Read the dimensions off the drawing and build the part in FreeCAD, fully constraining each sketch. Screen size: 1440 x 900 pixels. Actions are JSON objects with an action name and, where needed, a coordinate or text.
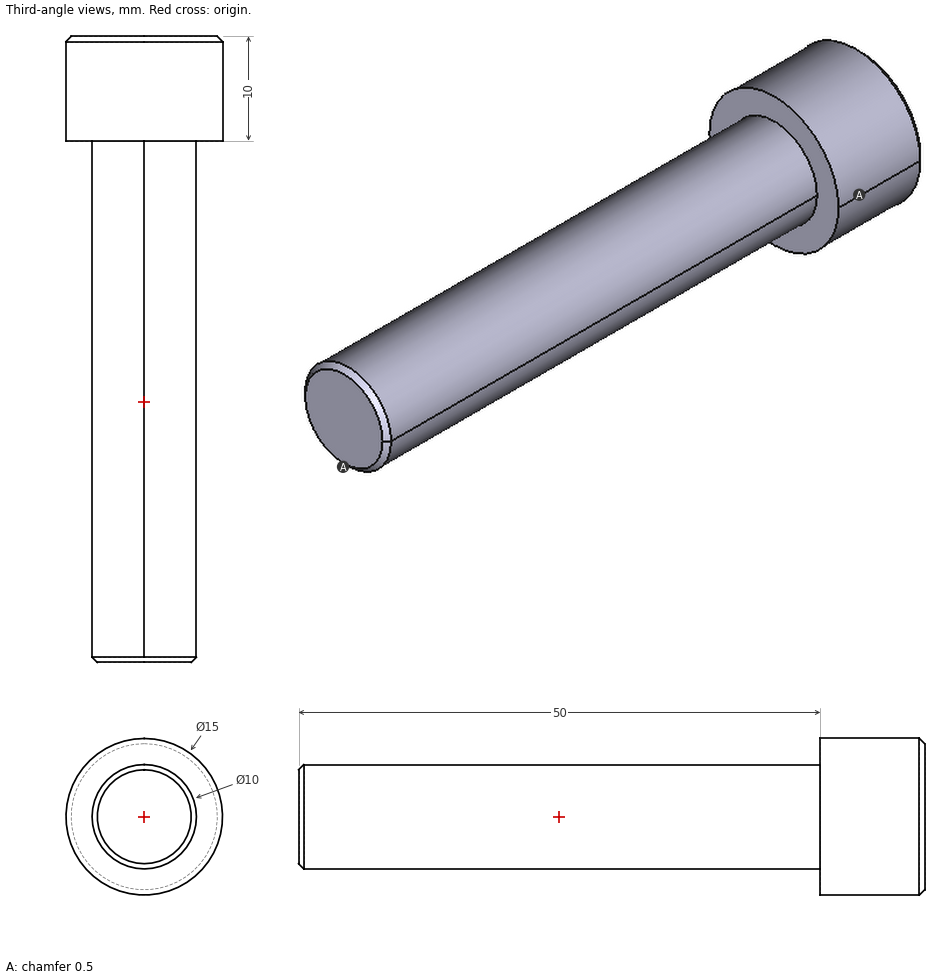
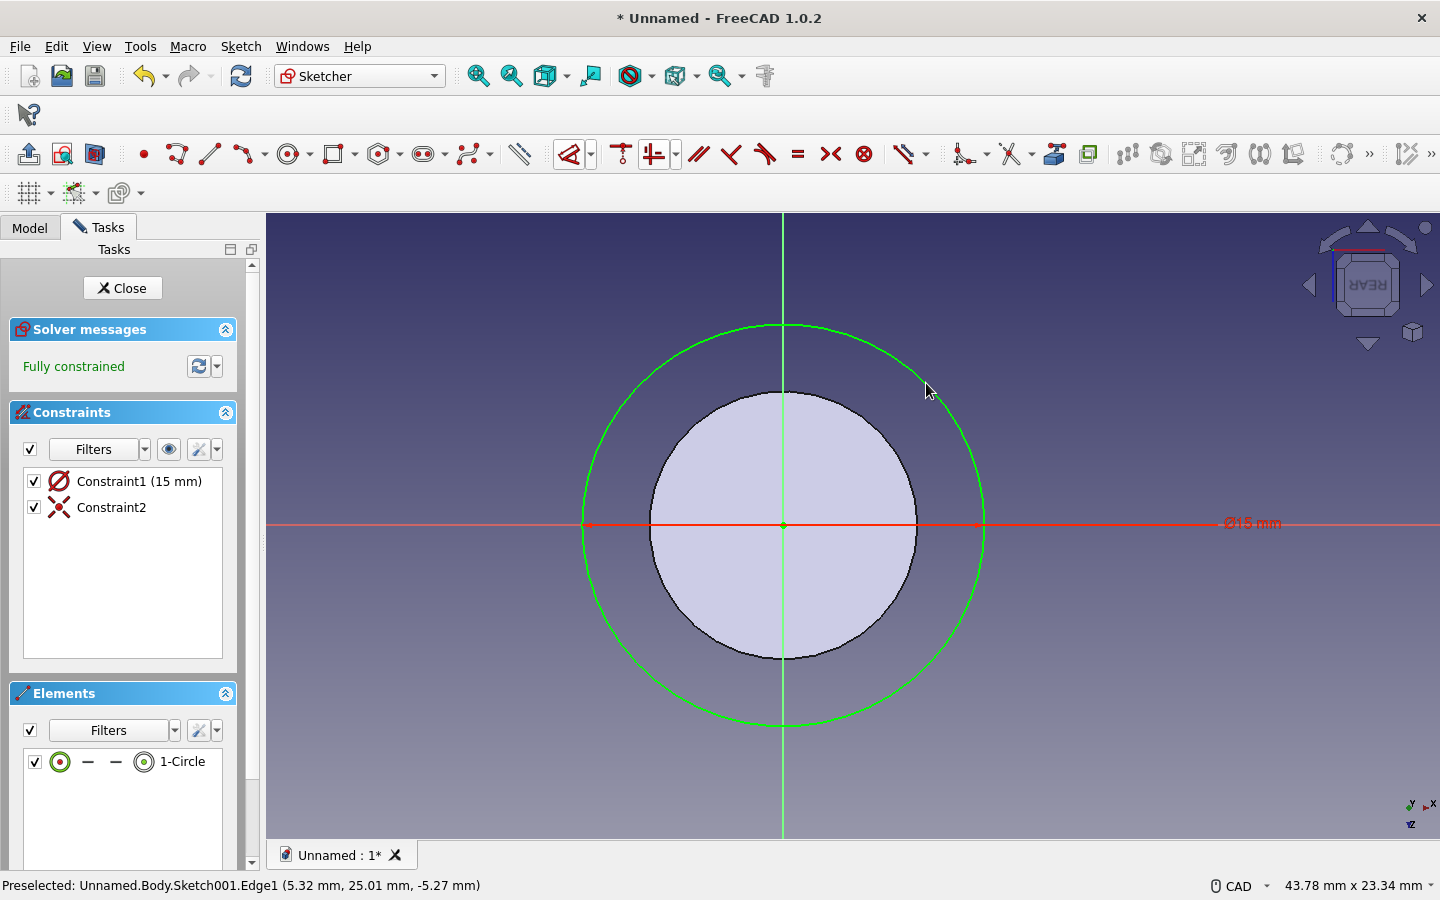
{"action": "left_click", "coordinate": [123, 288]}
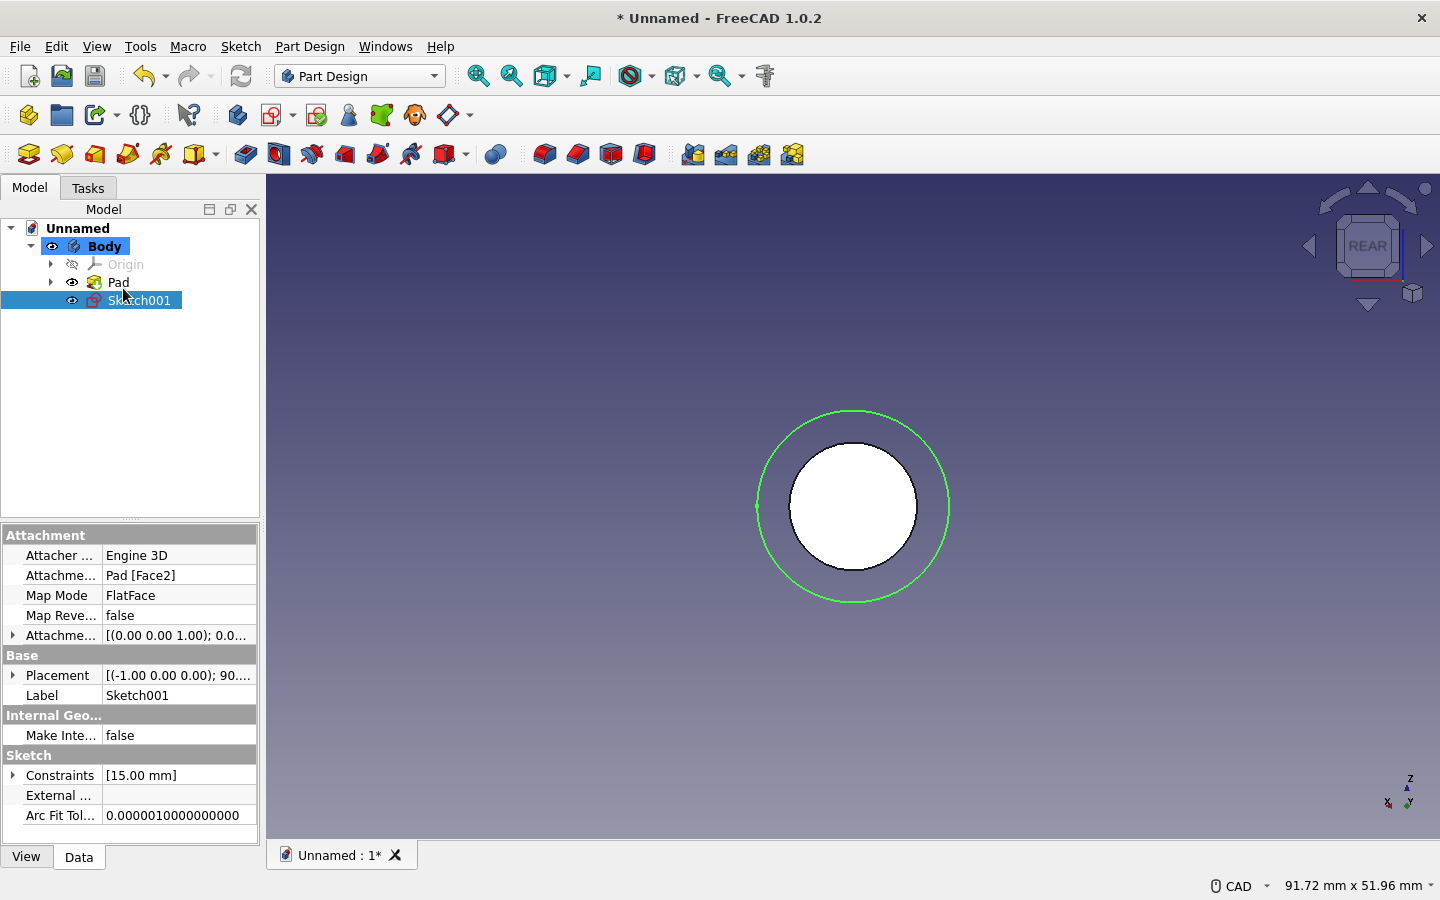
{"action": "left_click", "coordinate": [29, 154]}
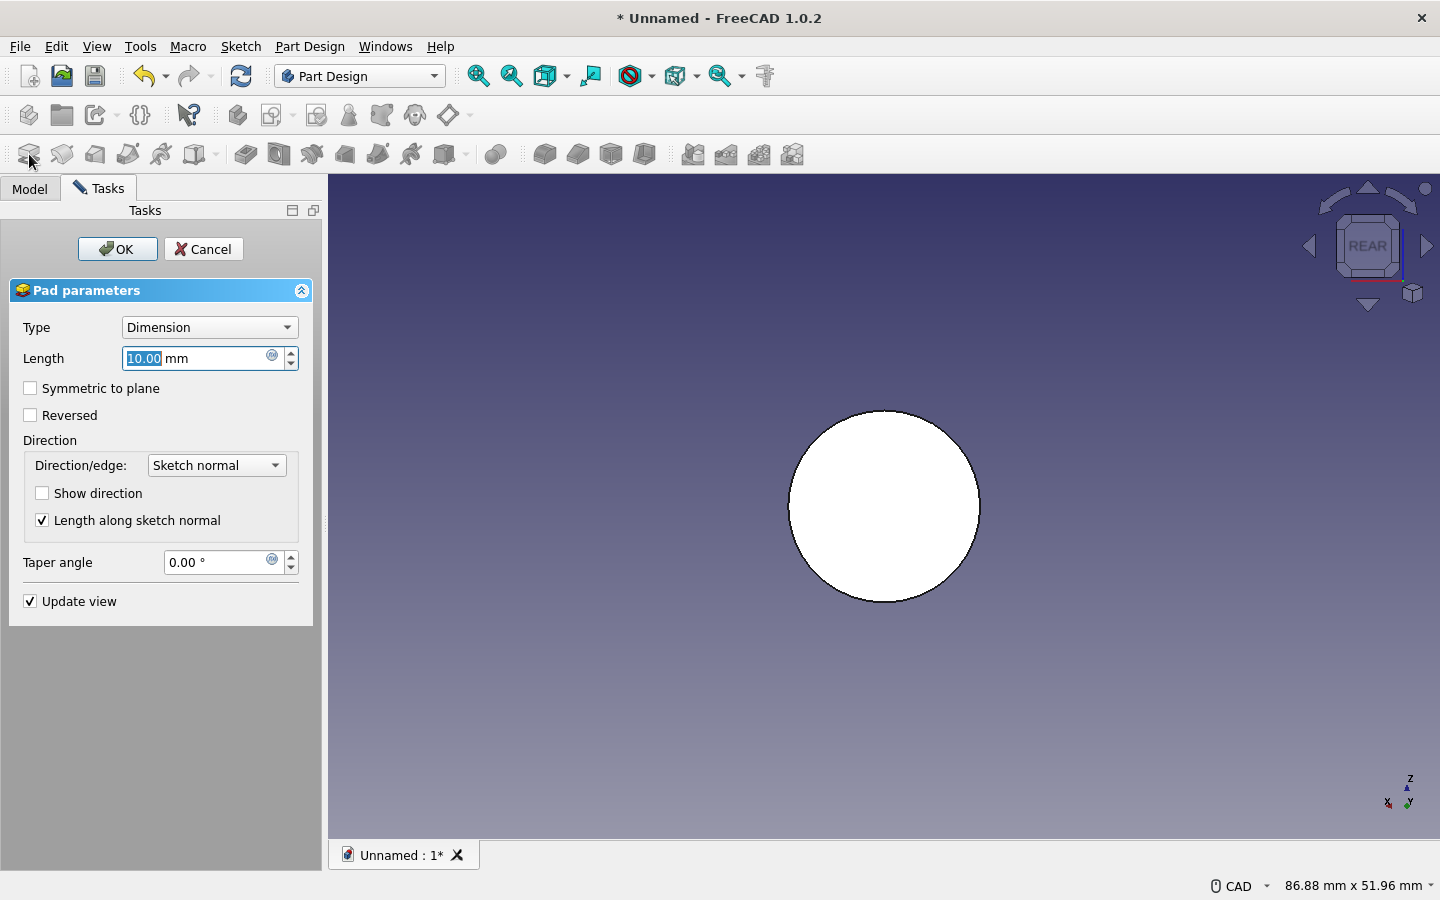
{"action": "type", "text": "10"}
{"action": "key", "text": "Tab"}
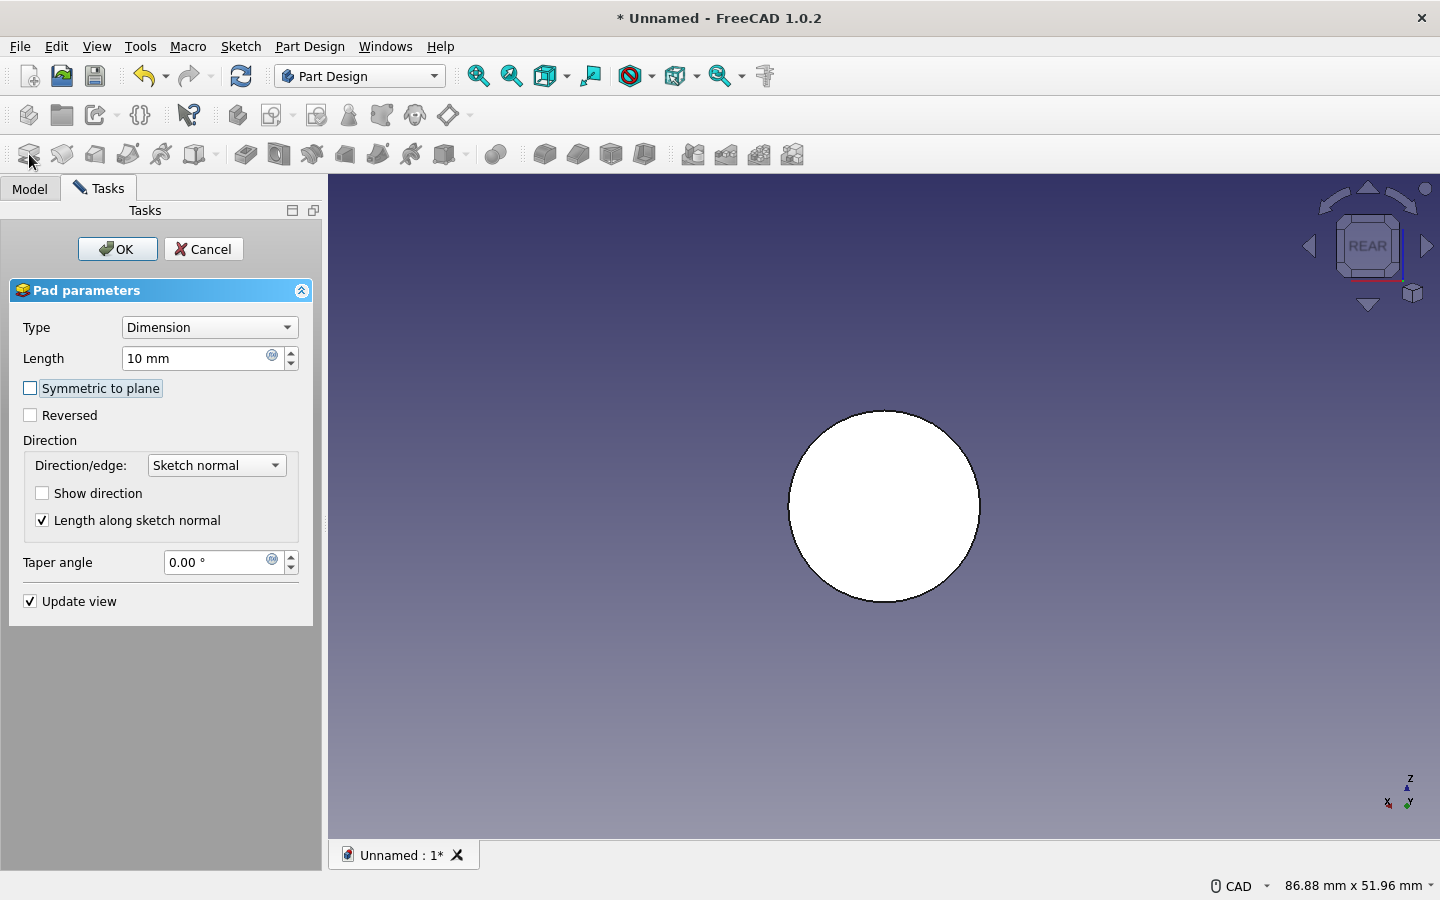
{"action": "left_click", "coordinate": [118, 249]}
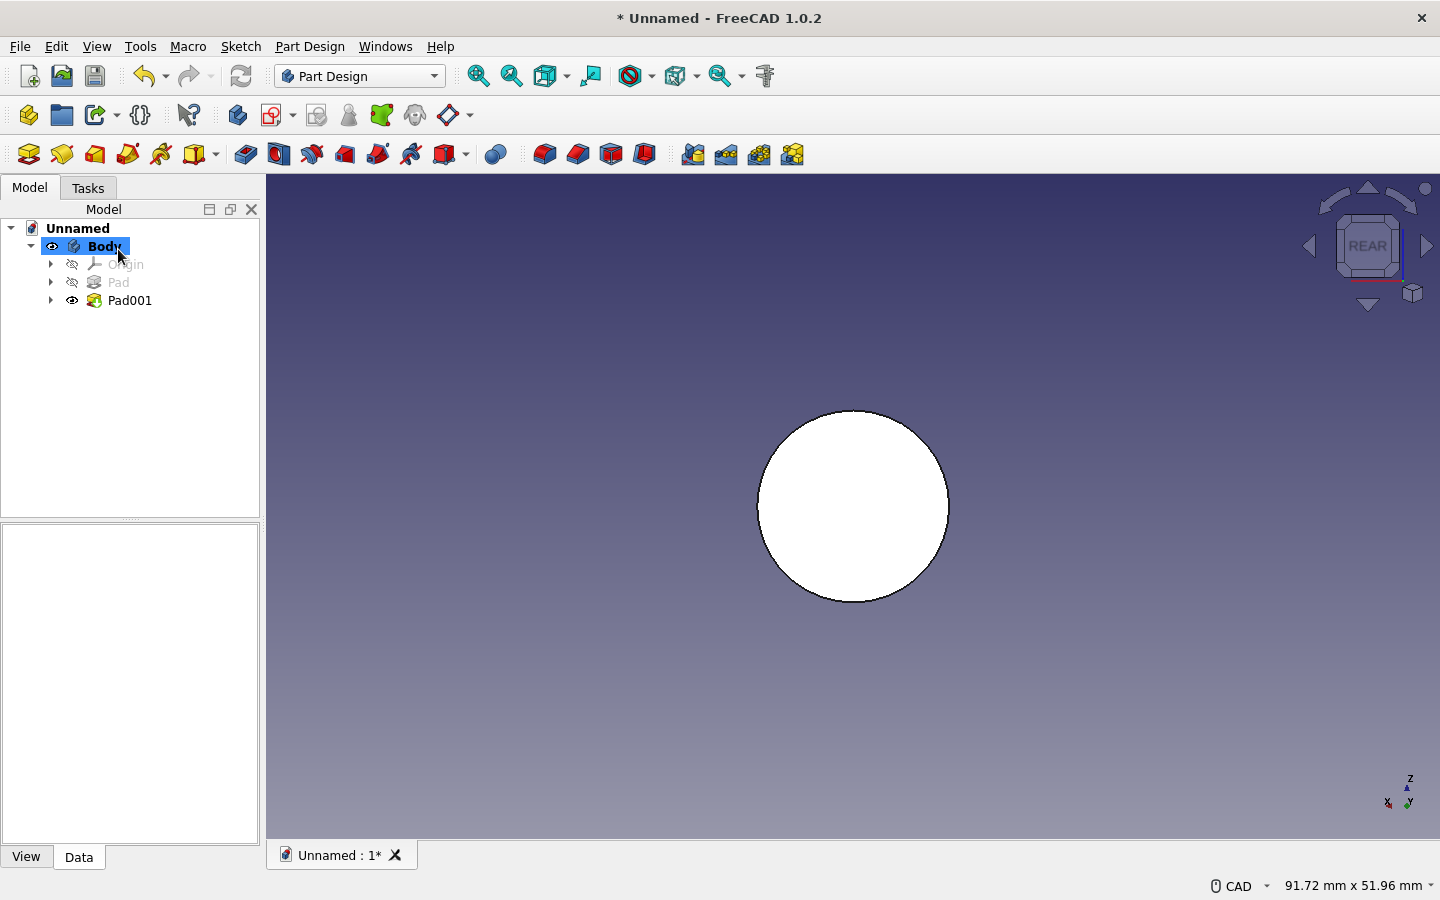
{"action": "key", "text": "v f"}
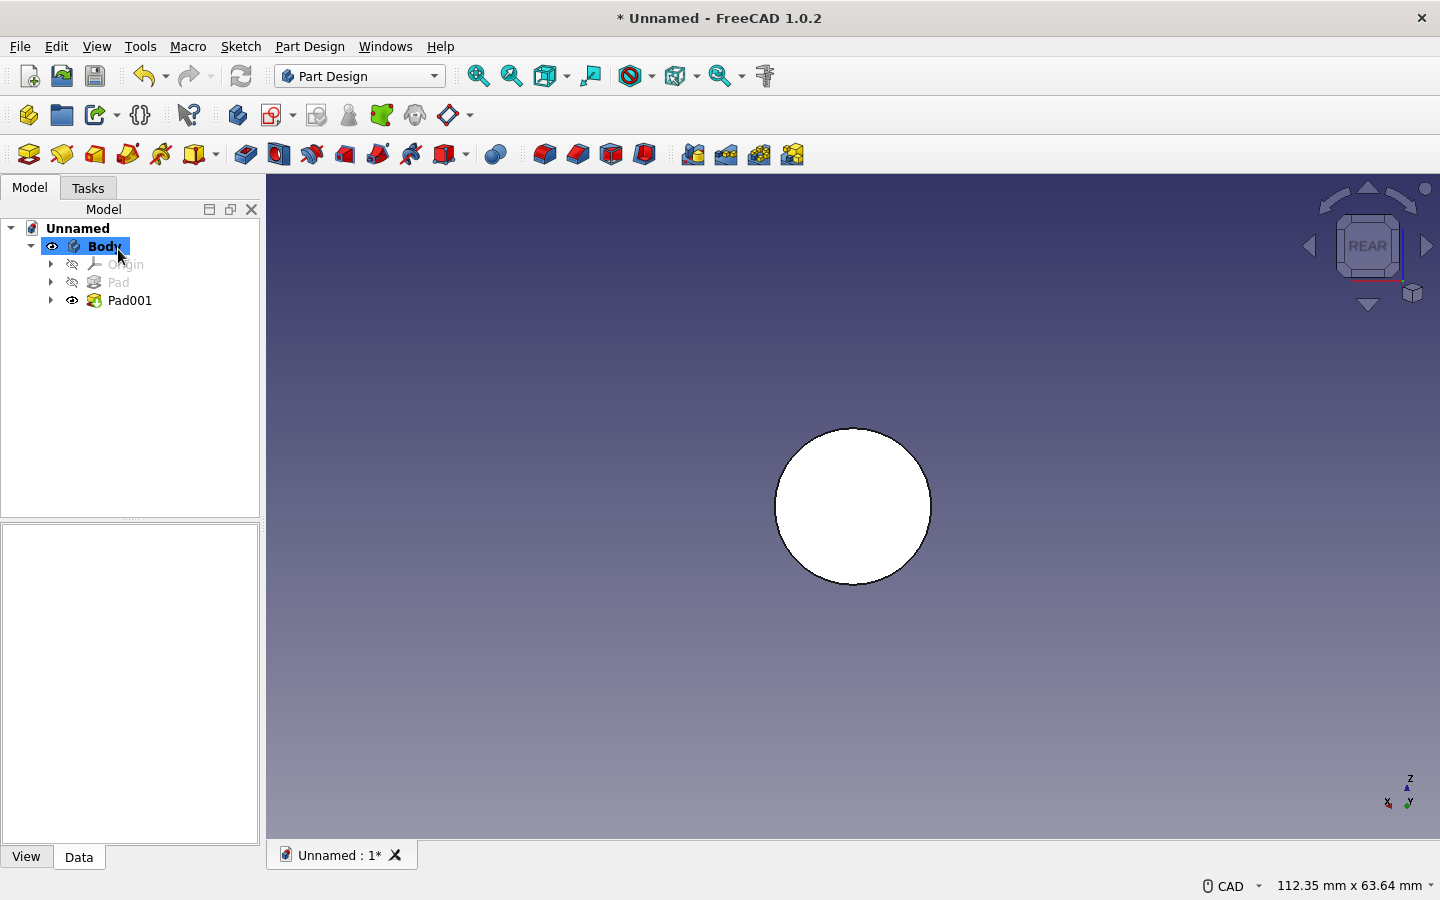
{"action": "left_click", "coordinate": [931, 505]}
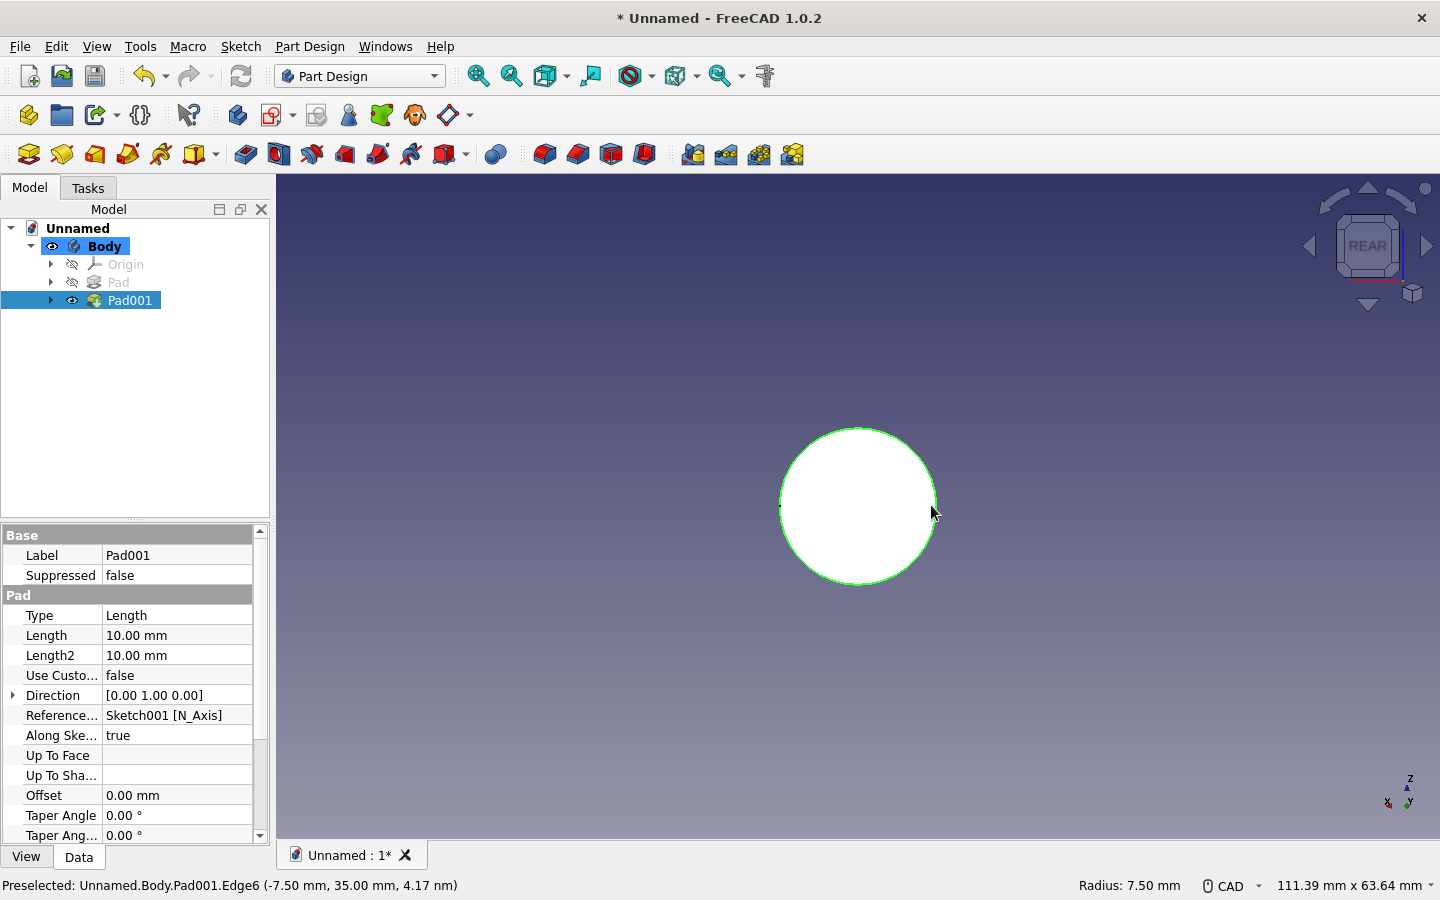
{"action": "key", "text": "0"}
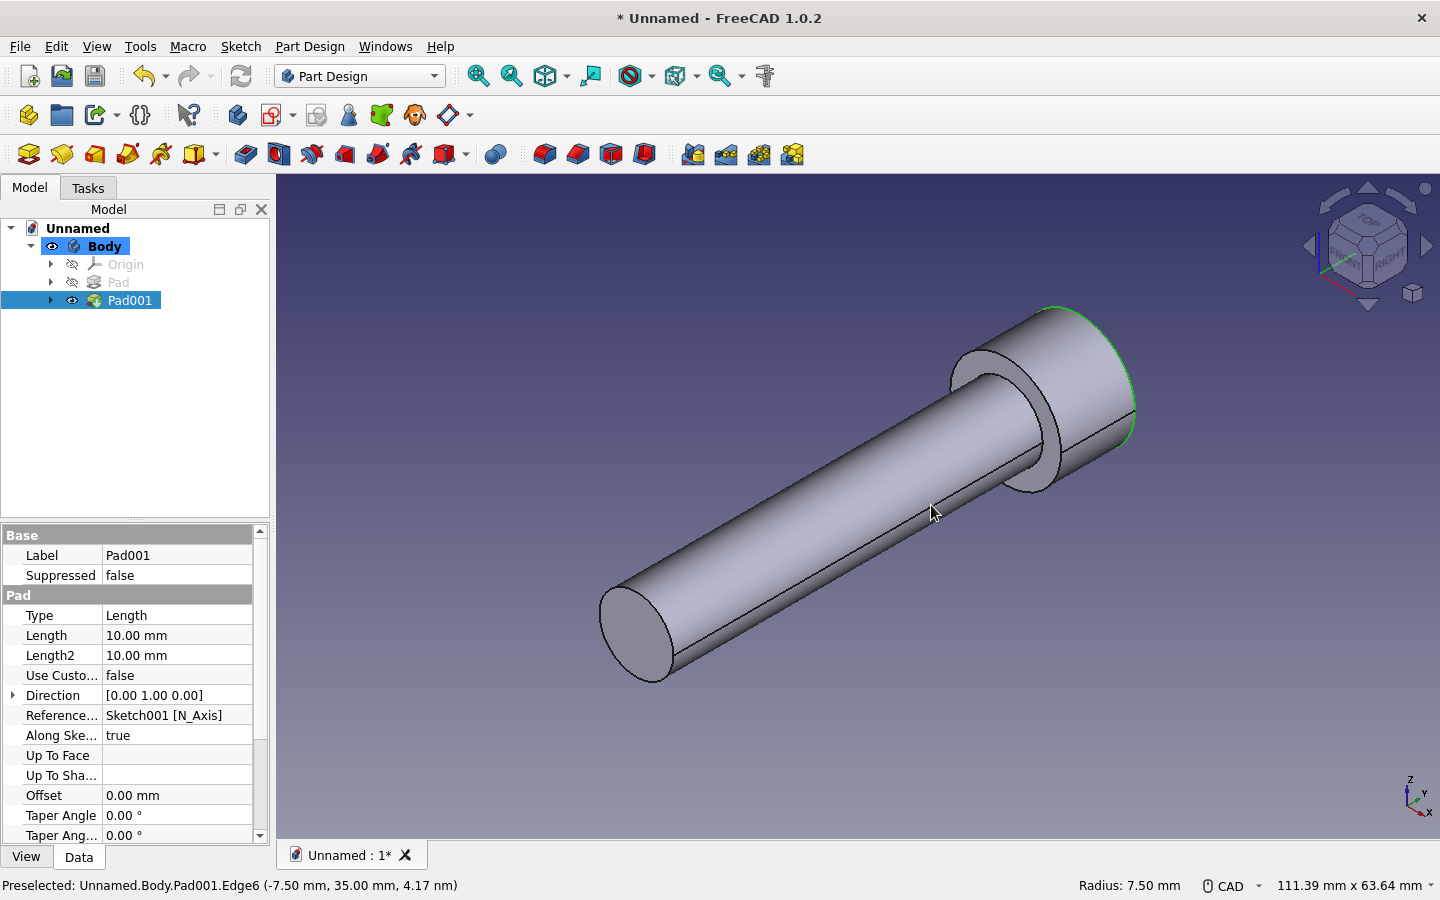
{"action": "left_click", "coordinate": [625, 586], "text": "ctrl"}